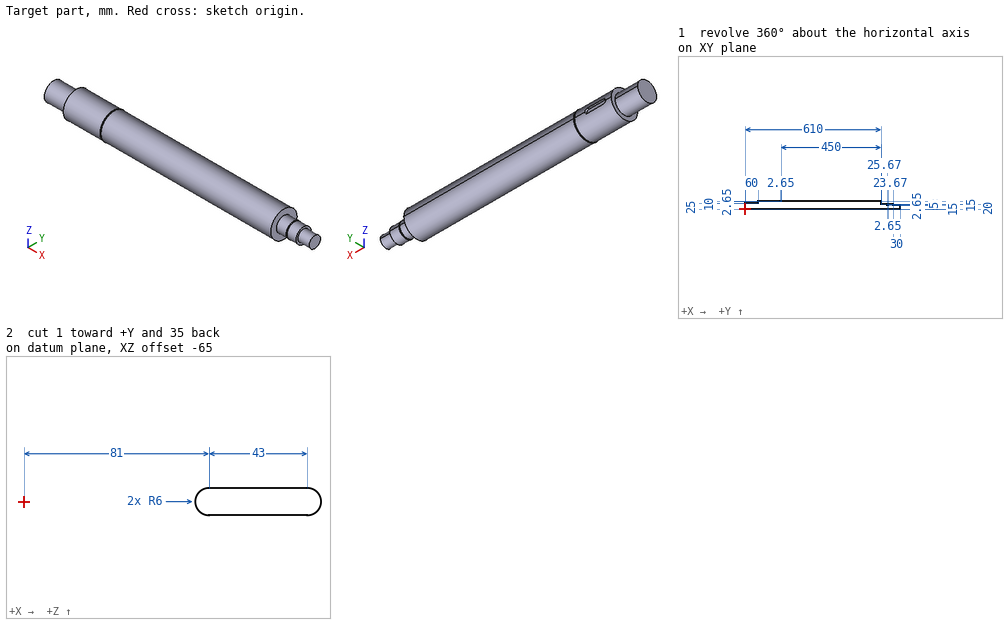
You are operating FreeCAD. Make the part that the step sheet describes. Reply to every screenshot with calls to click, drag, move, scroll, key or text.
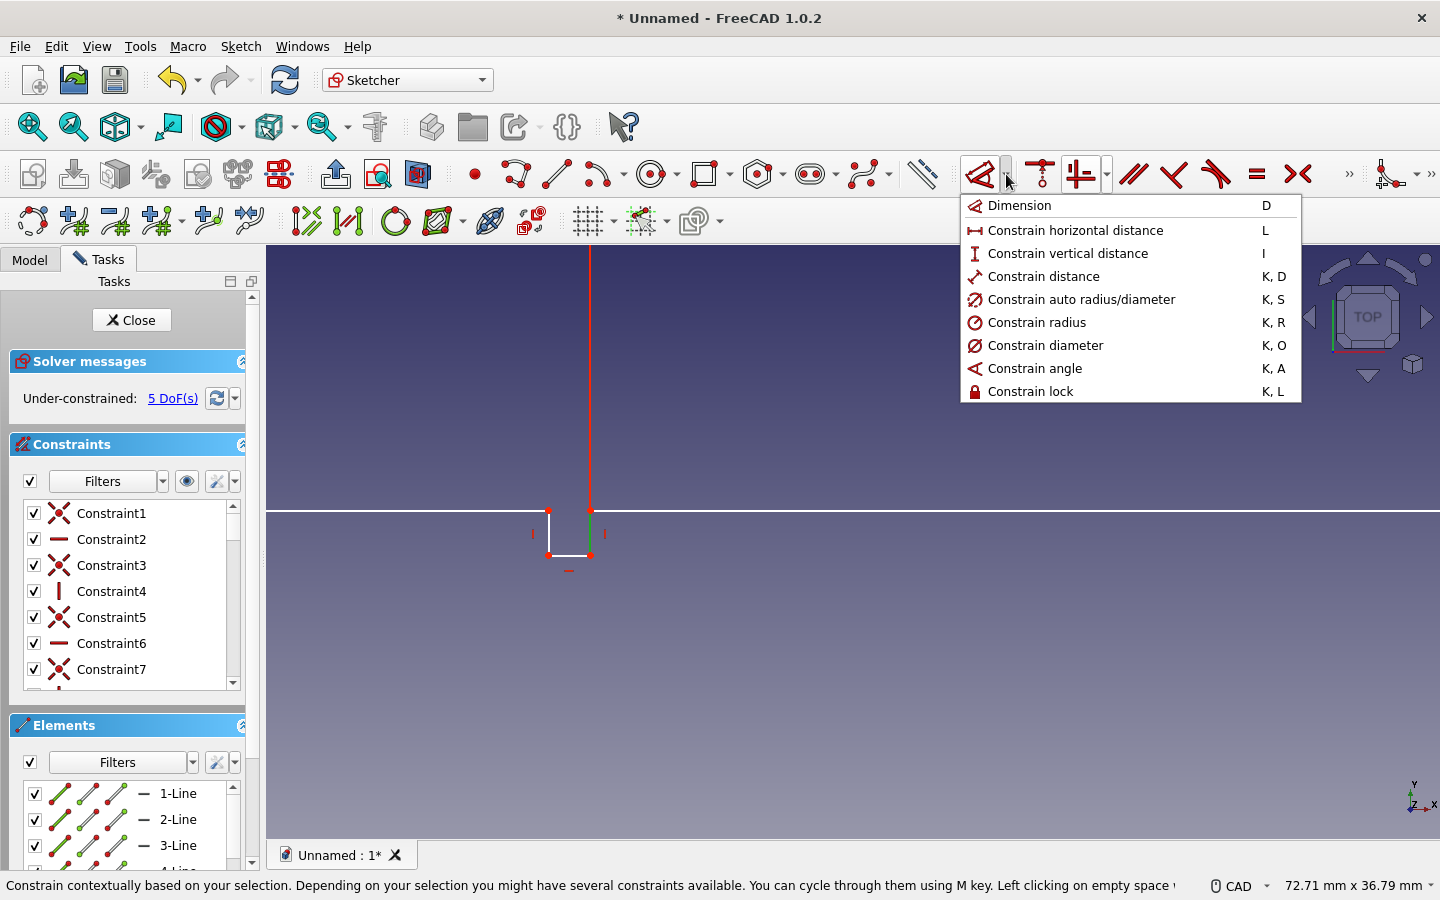
click(1131, 254)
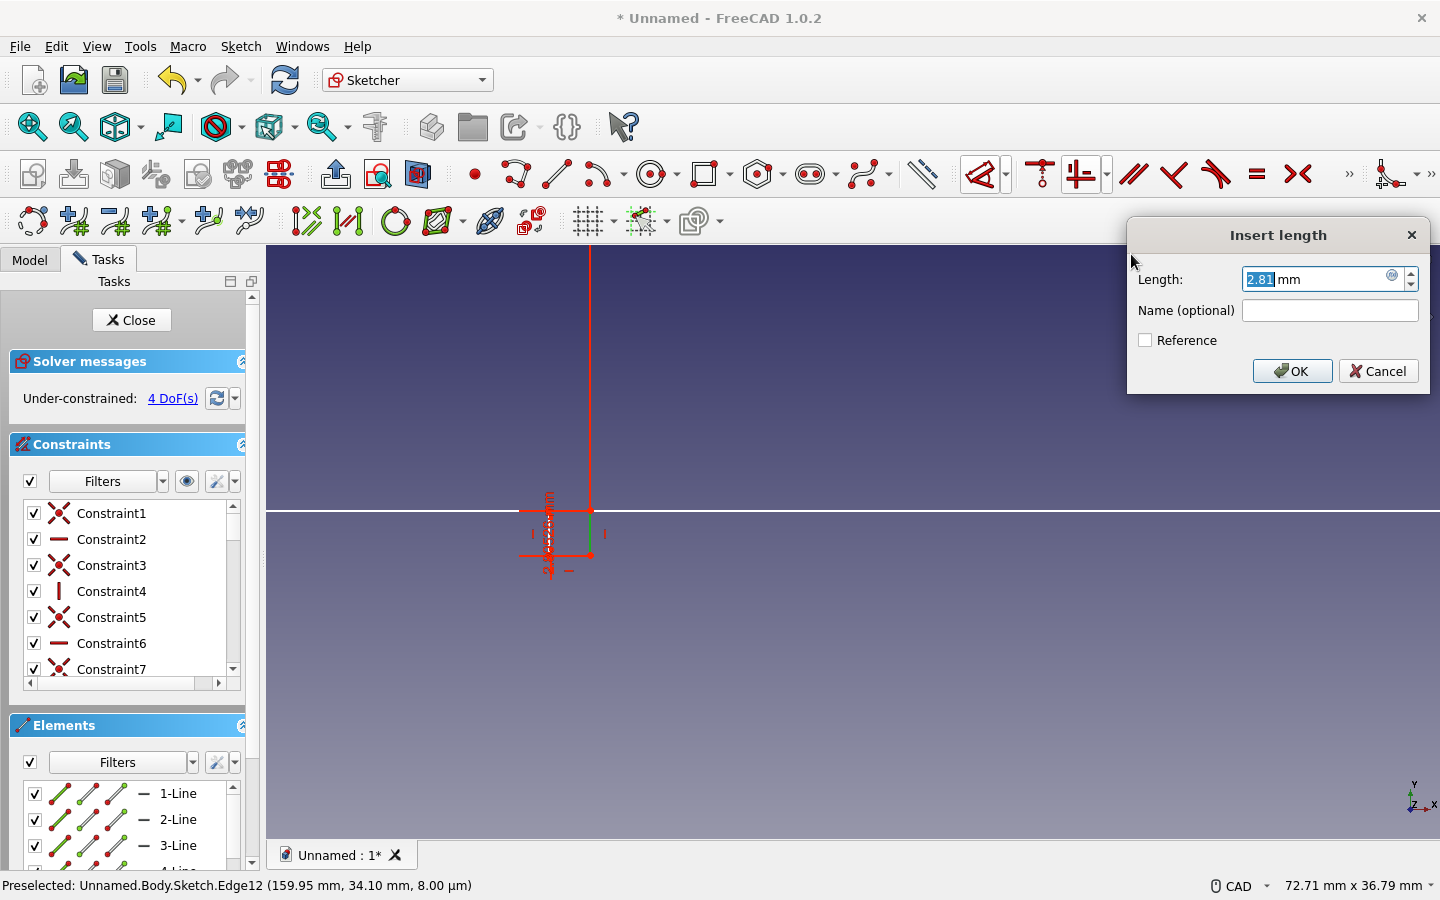
text(2.65)
key(Return)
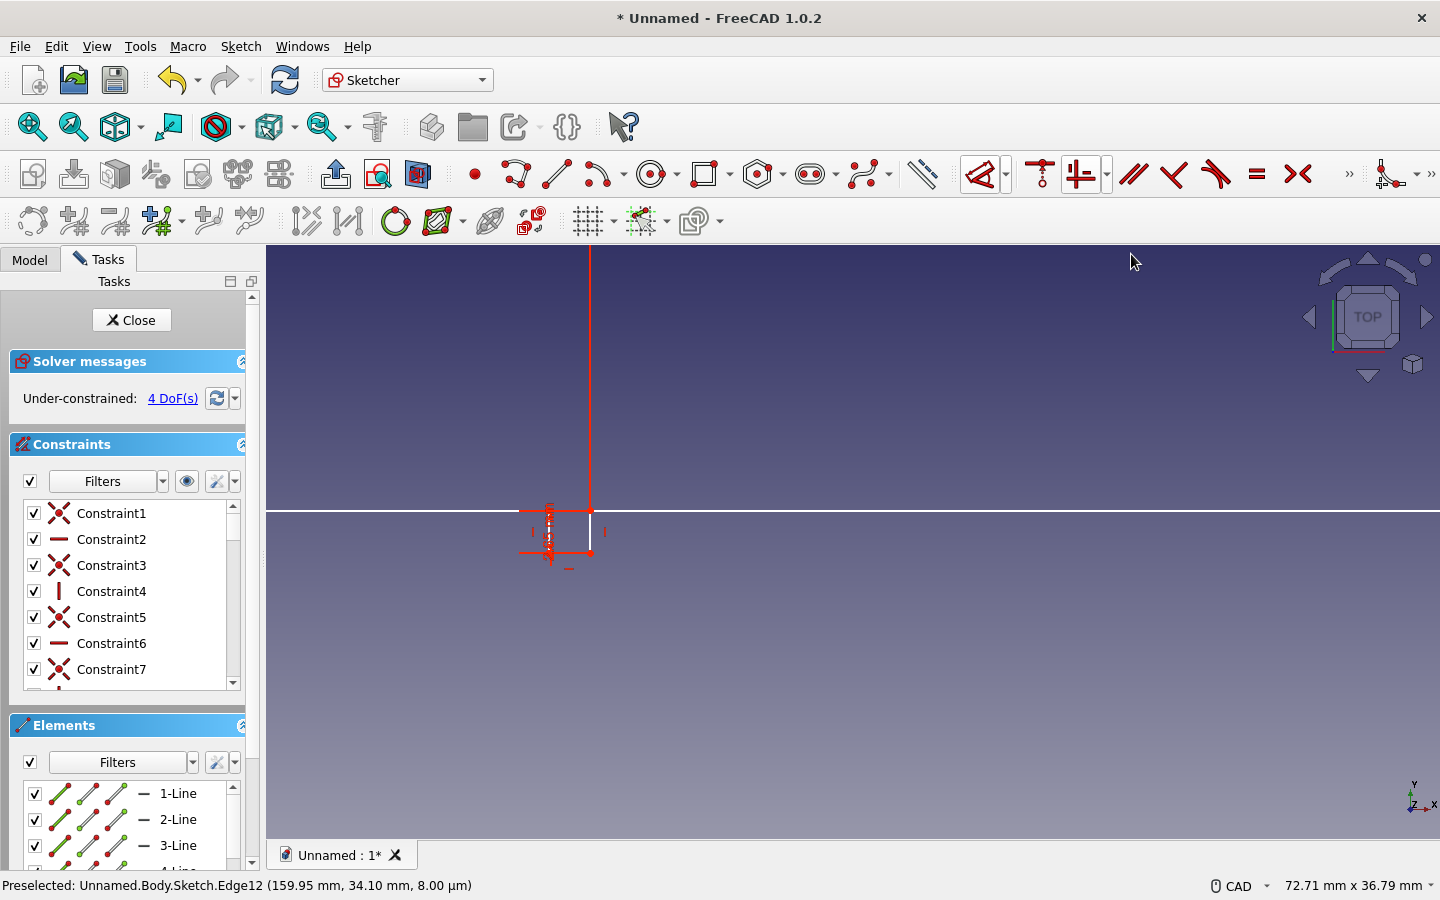
click(578, 553)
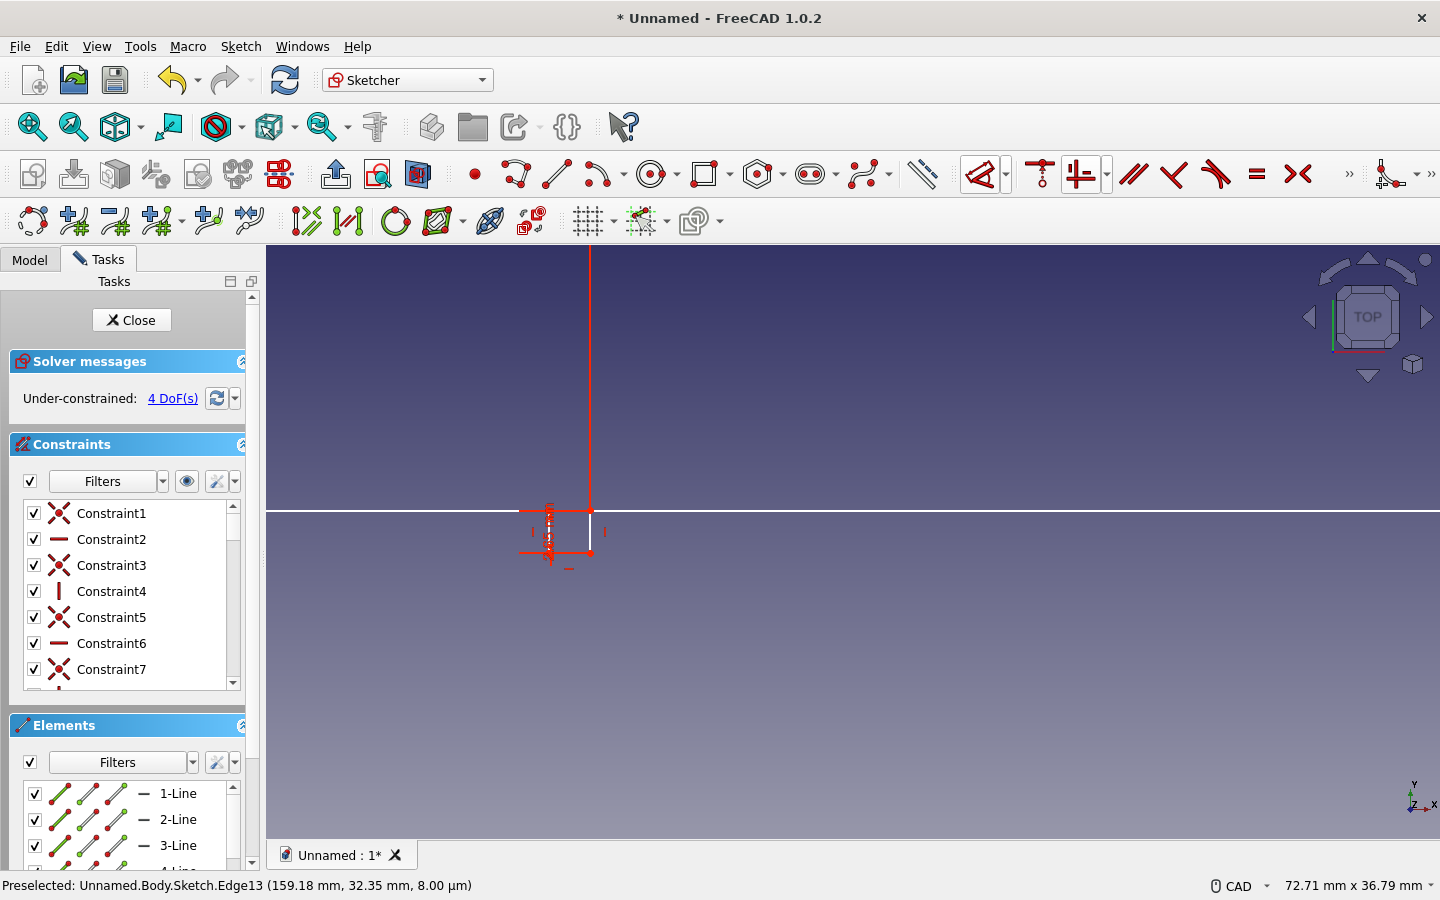
key(l)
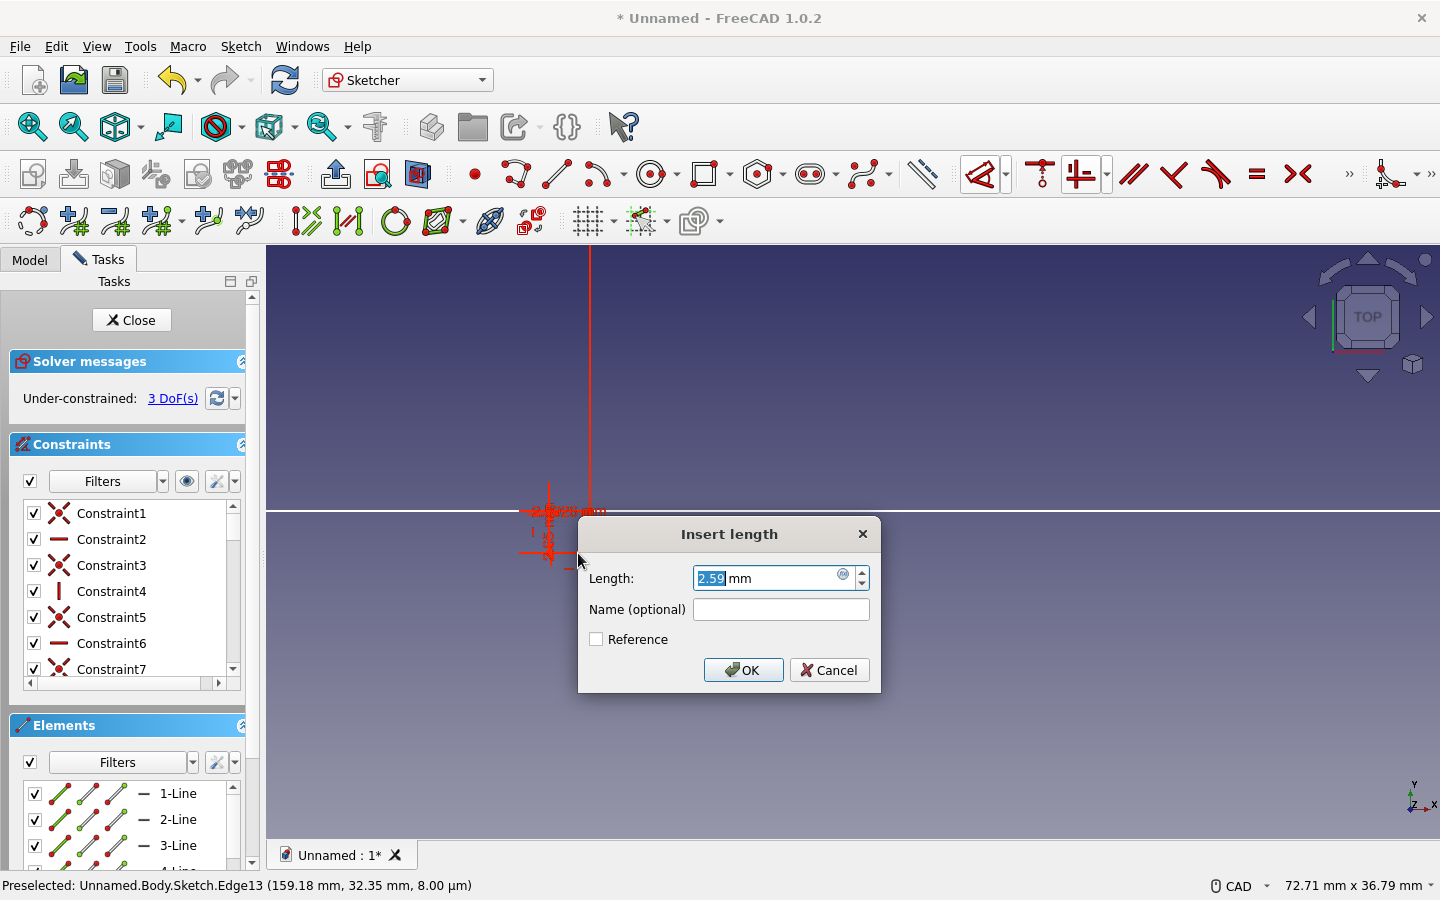
text(2.65)
key(Return)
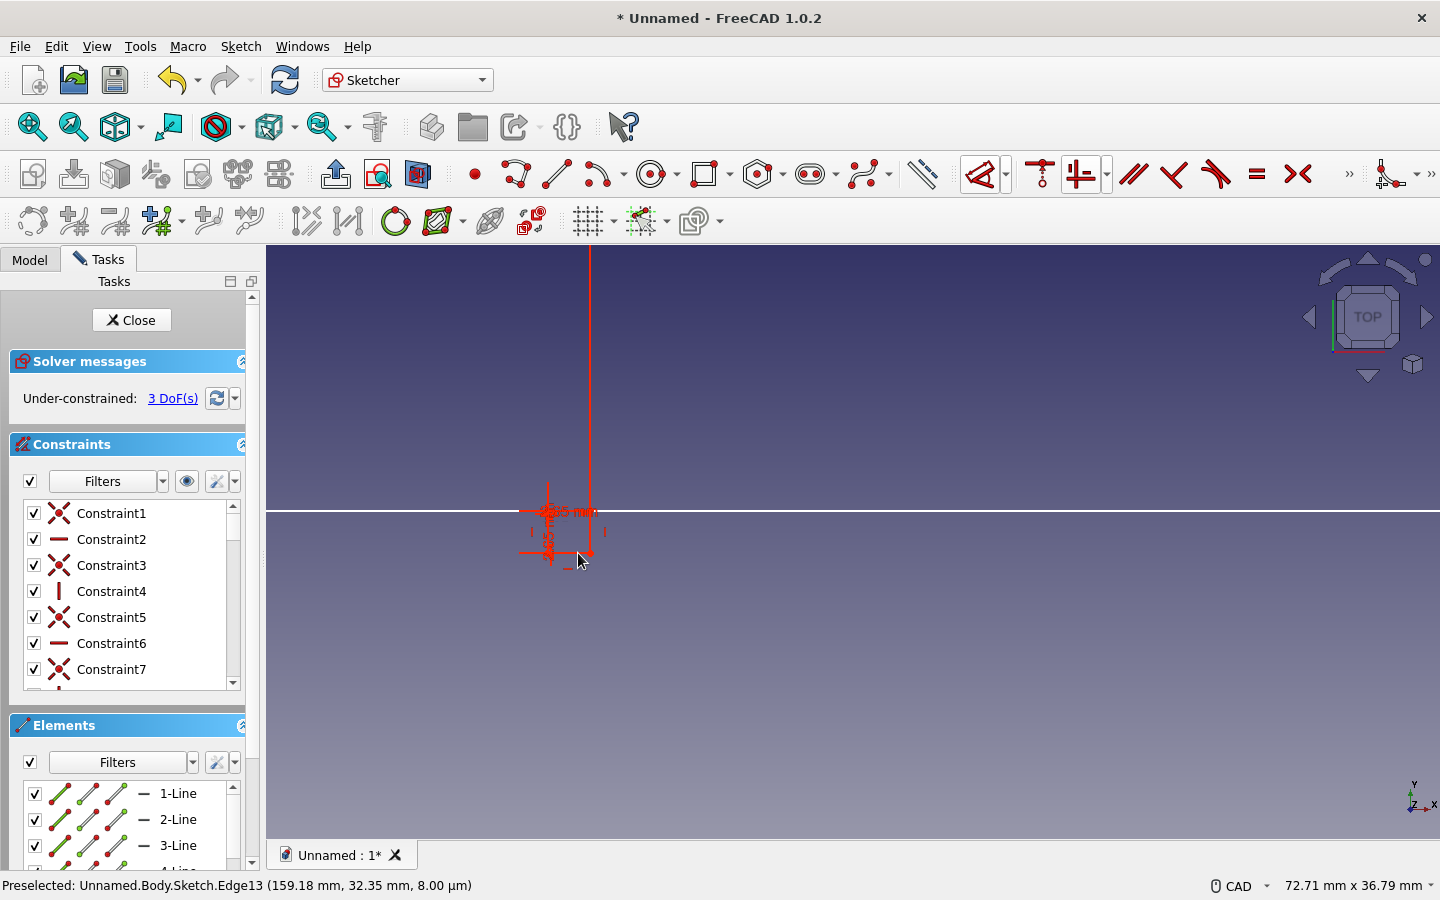
scroll(603, 526, down, 14)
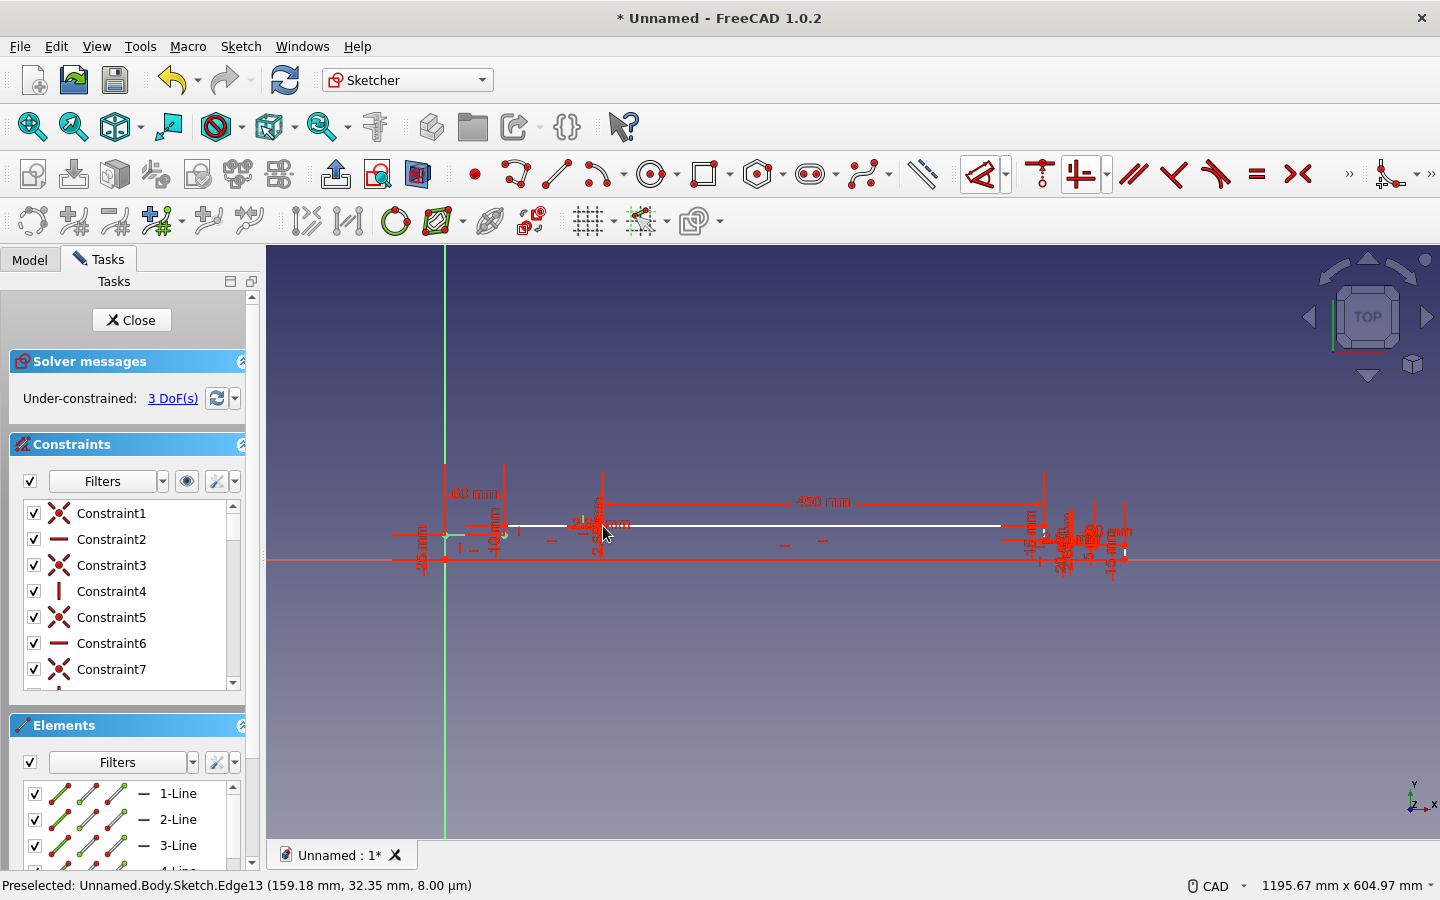
click(1044, 540)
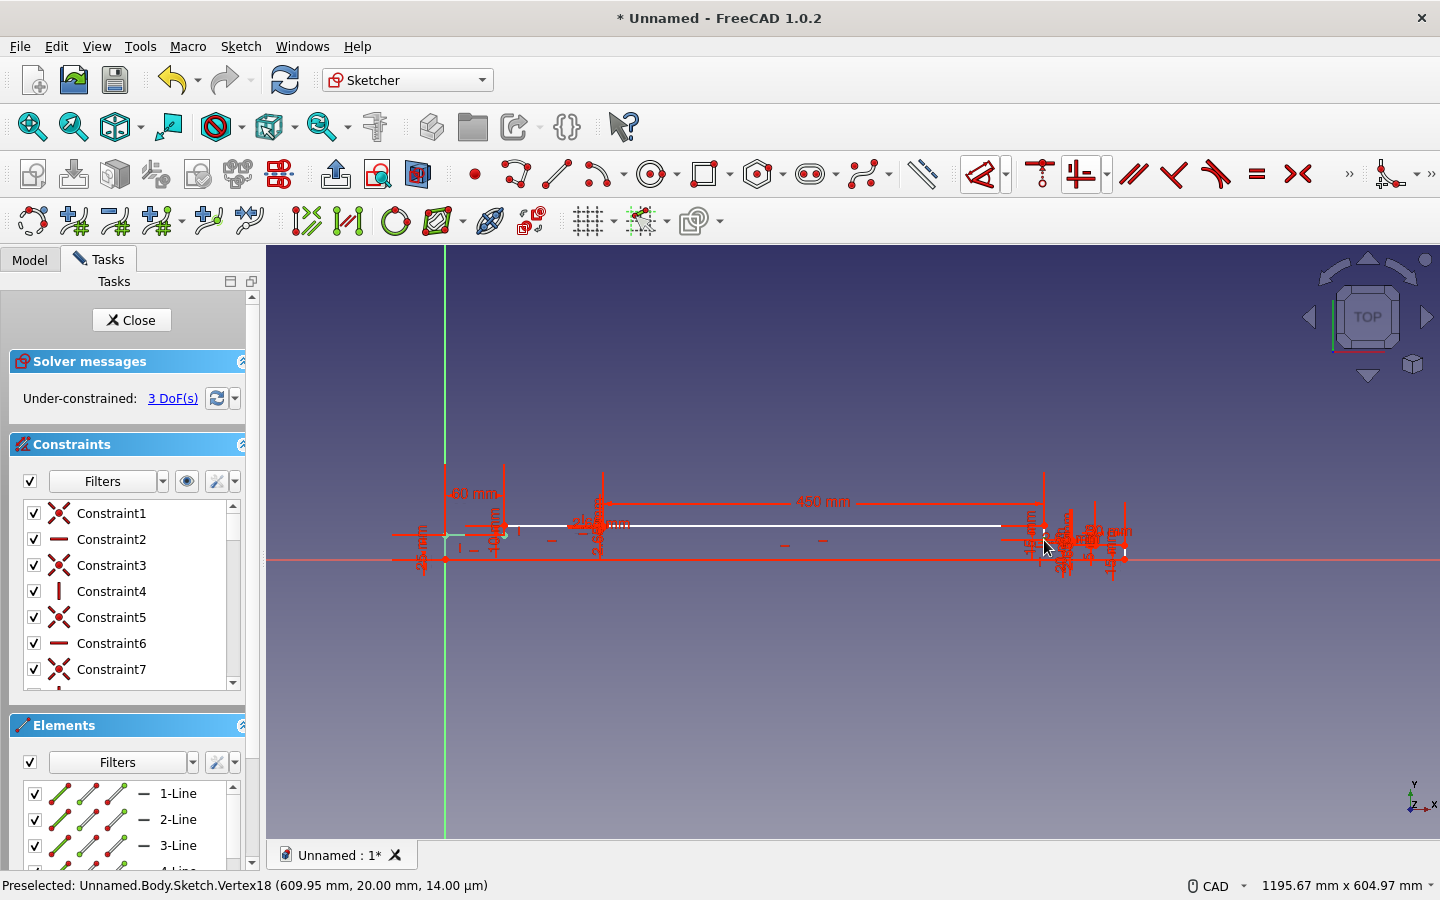
click(1006, 174)